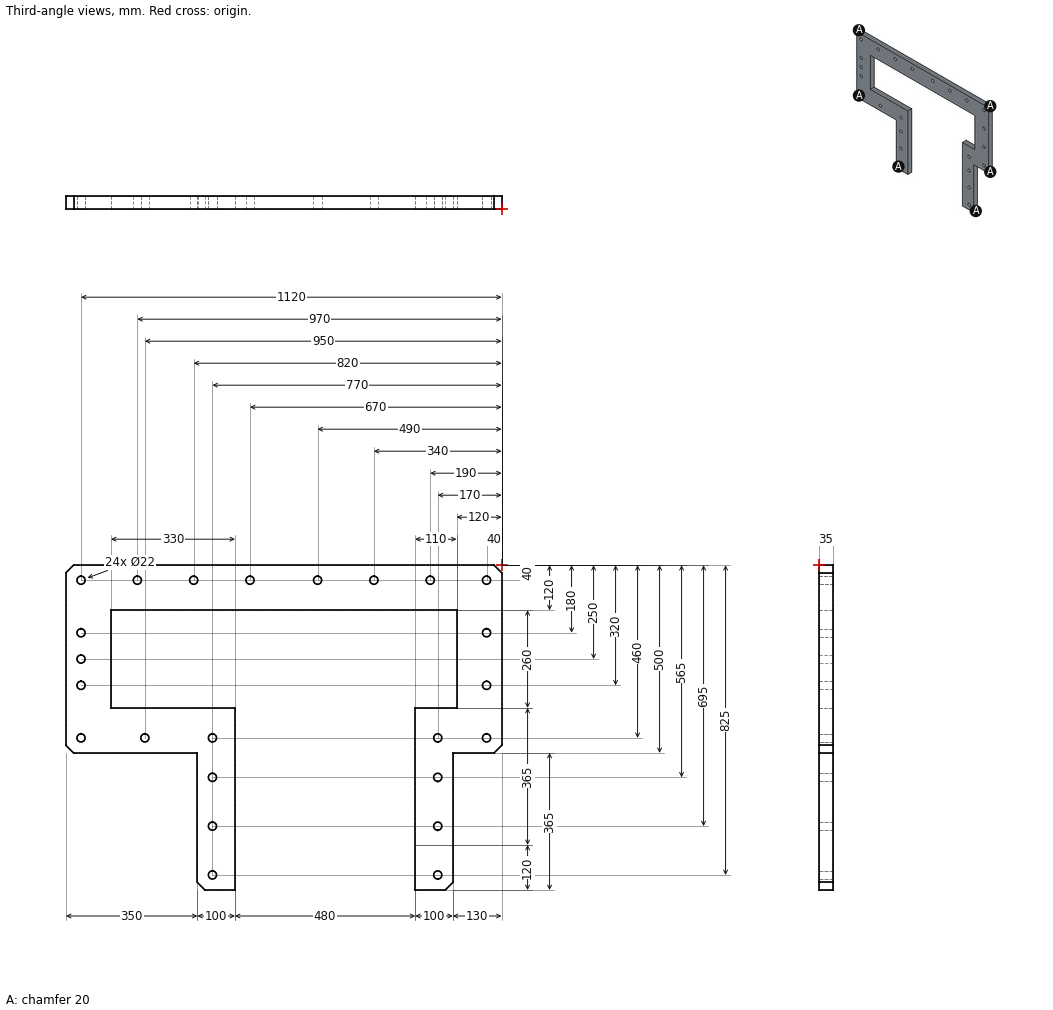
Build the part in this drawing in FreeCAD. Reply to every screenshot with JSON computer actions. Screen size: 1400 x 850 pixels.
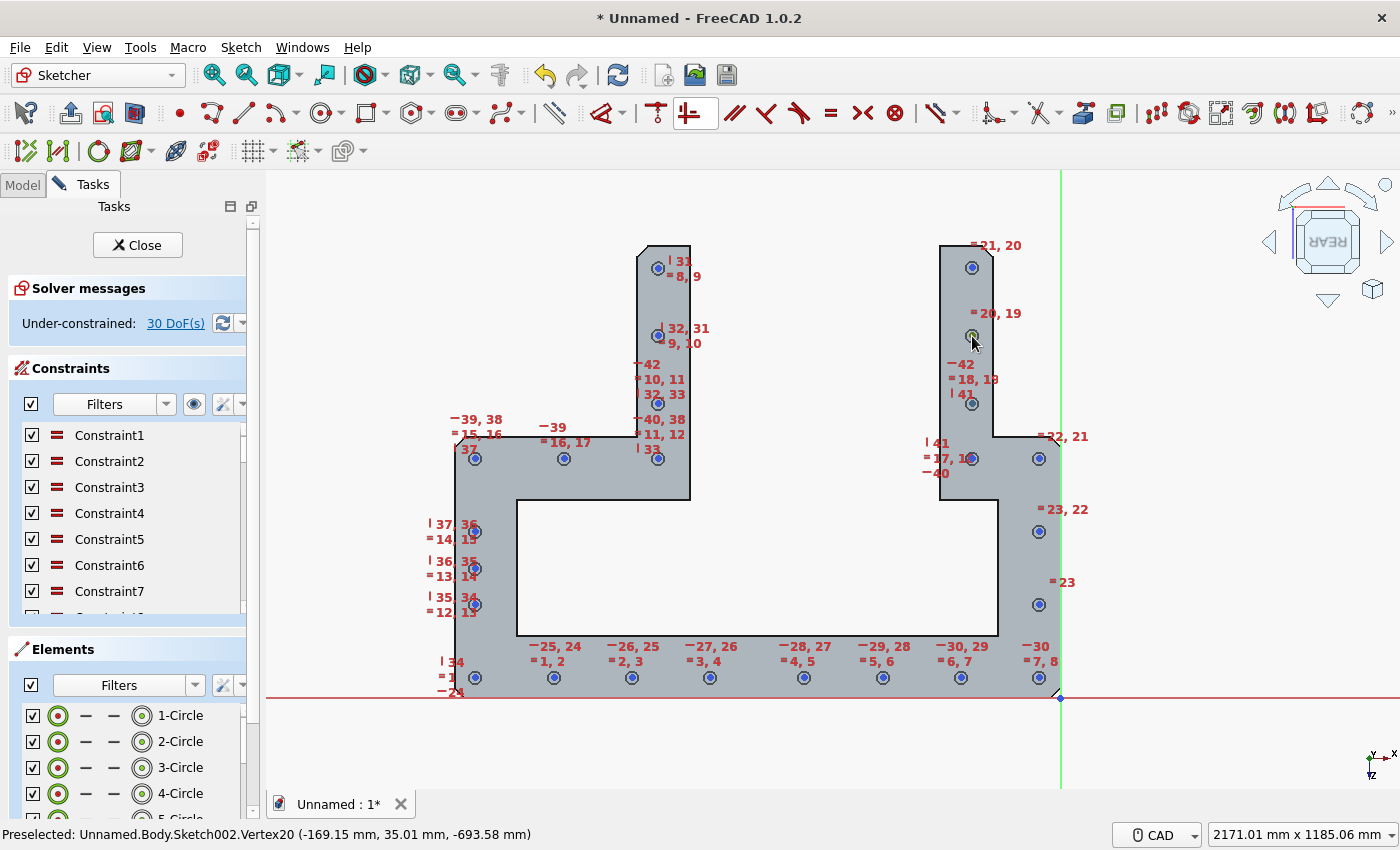
{"action": "key", "text": "v"}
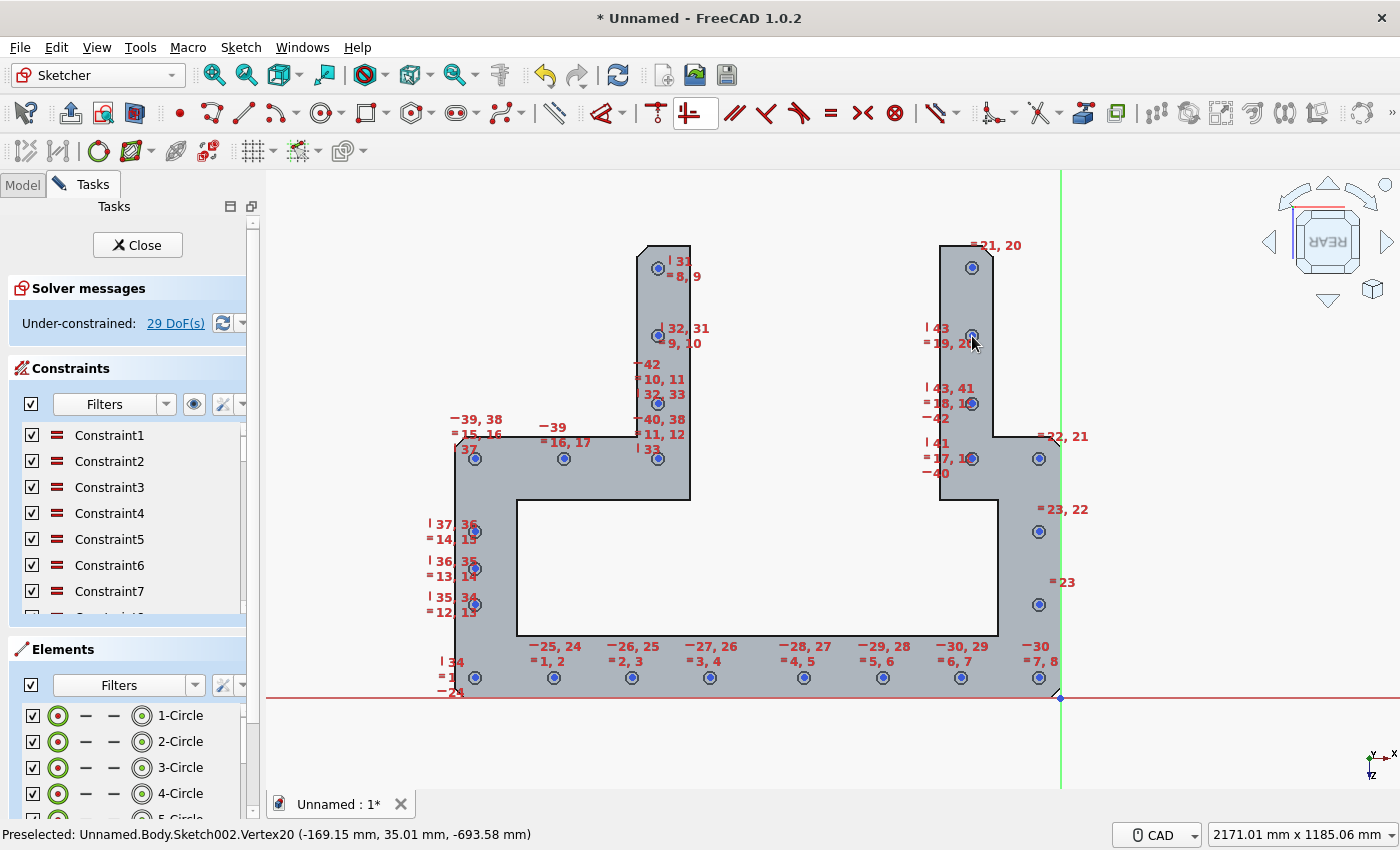
{"action": "left_click", "coordinate": [658, 336]}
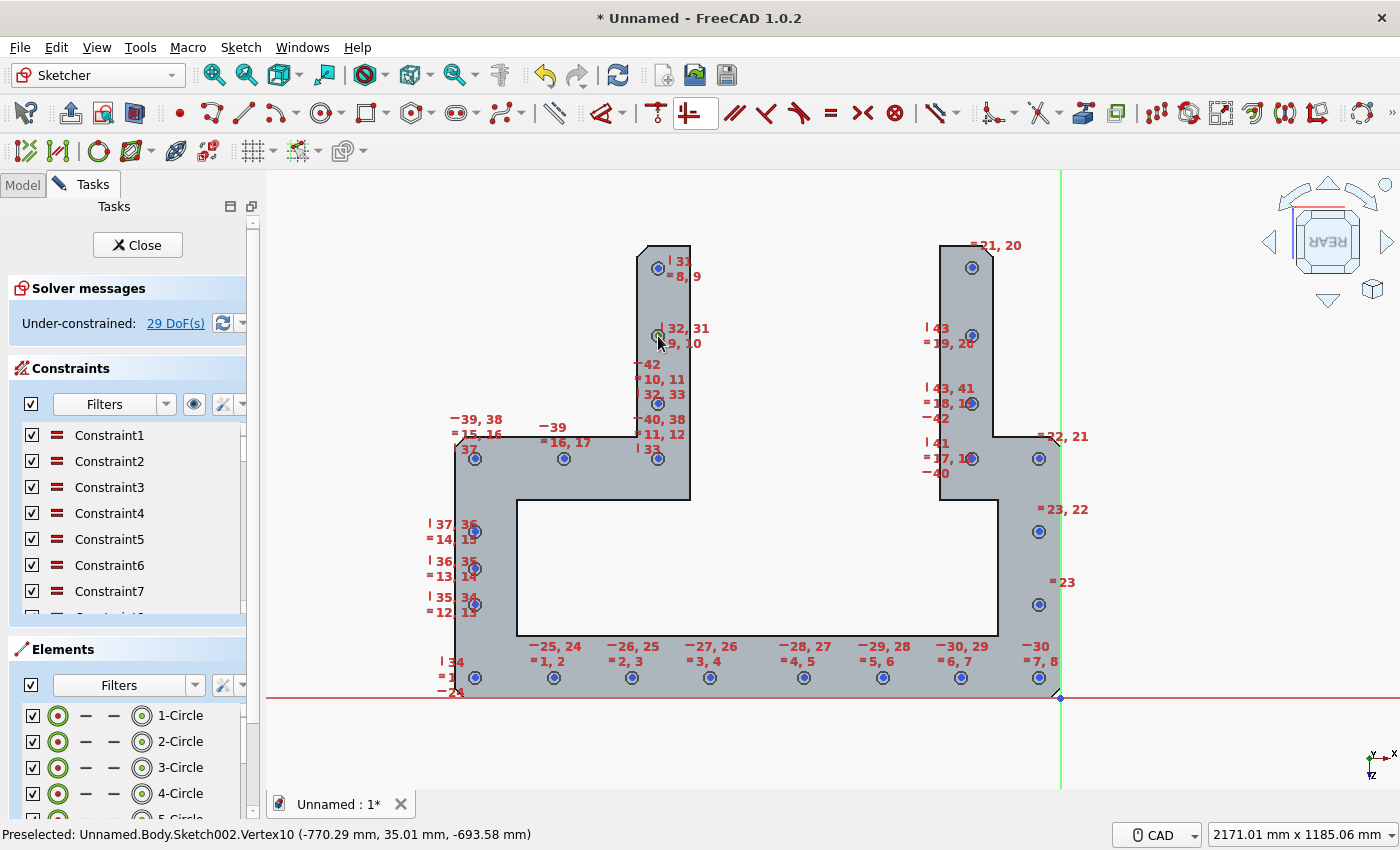
{"action": "left_click", "coordinate": [974, 338]}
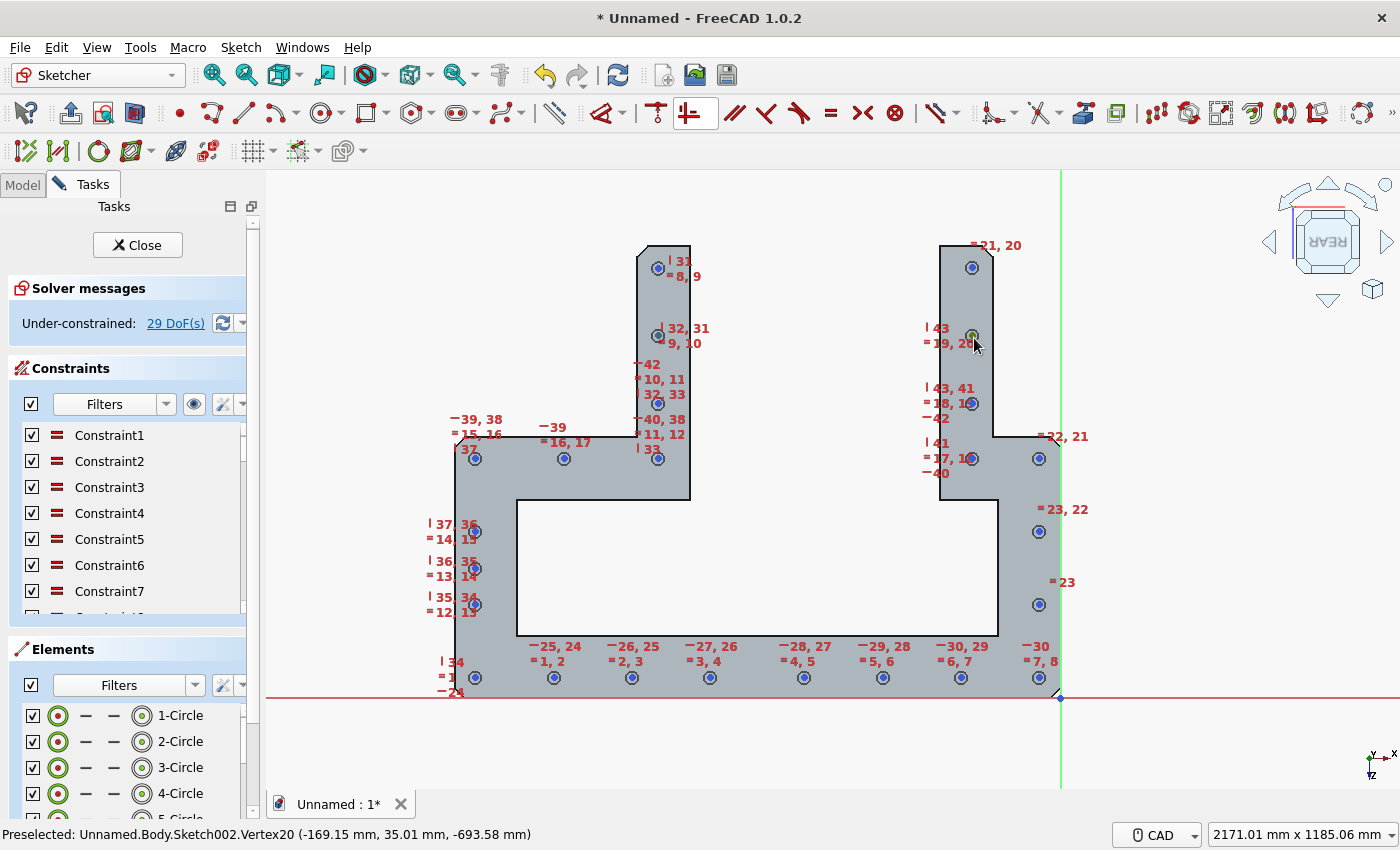
{"action": "key", "text": "h"}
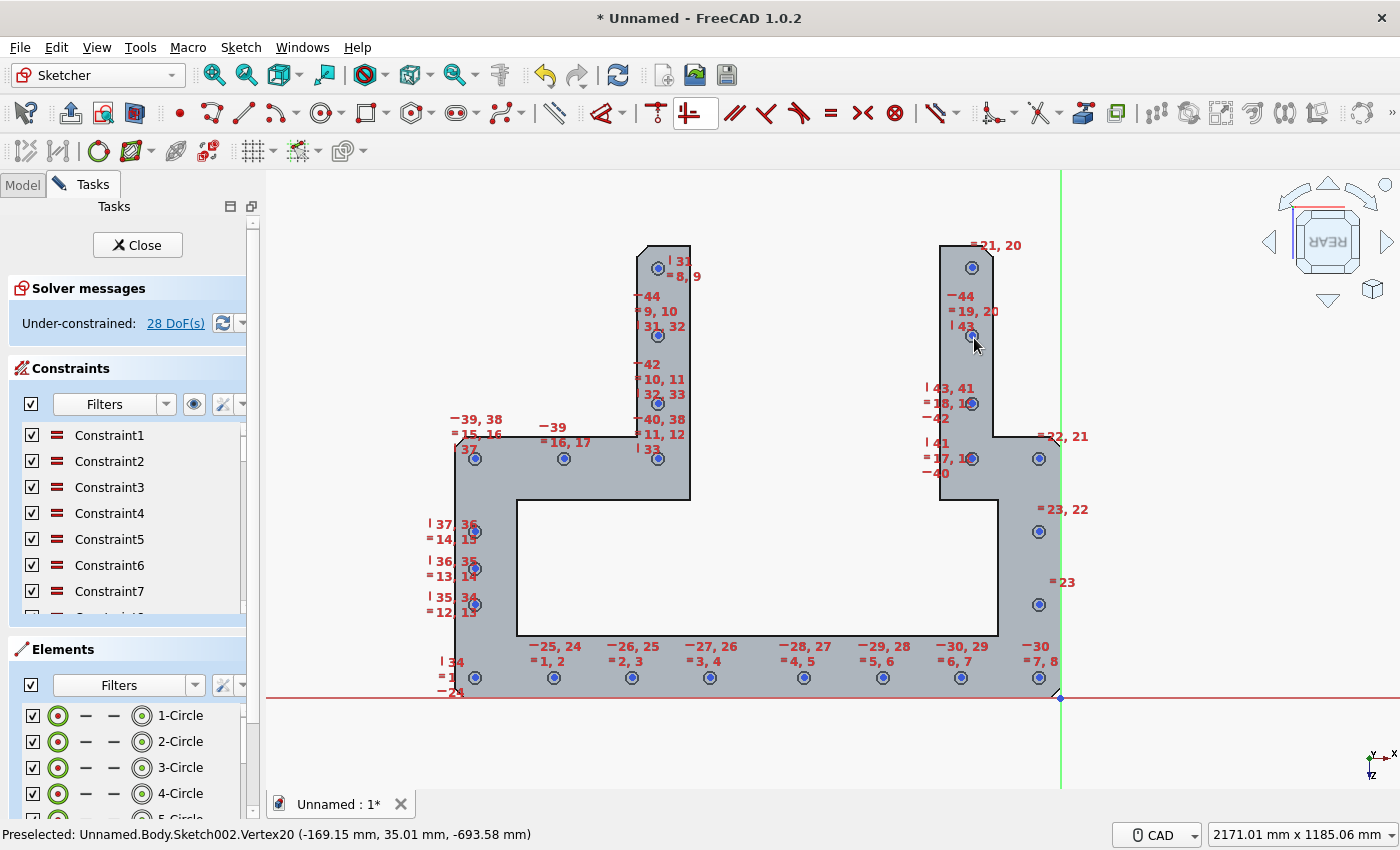
{"action": "left_click", "coordinate": [972, 336]}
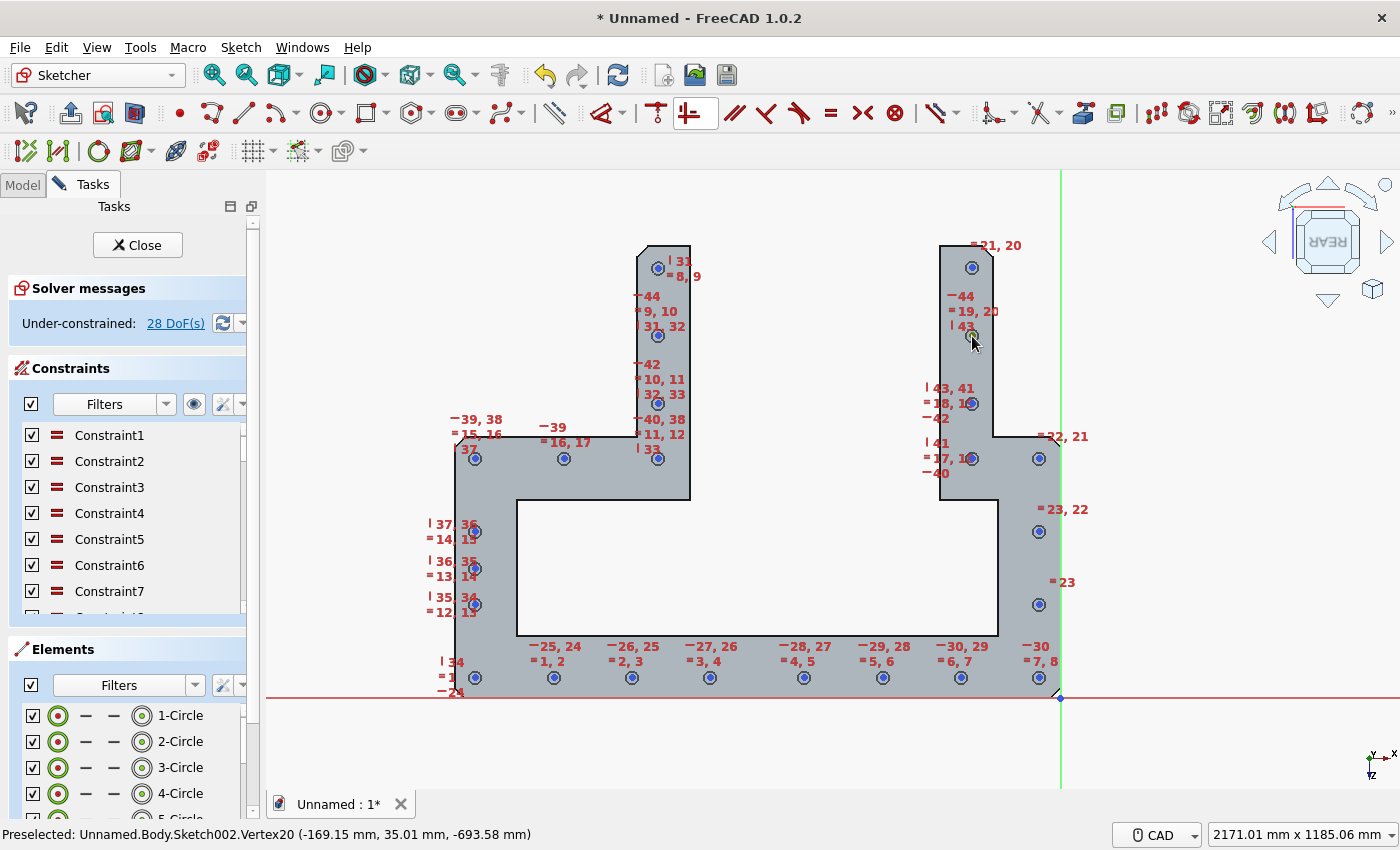
{"action": "left_click", "coordinate": [972, 268]}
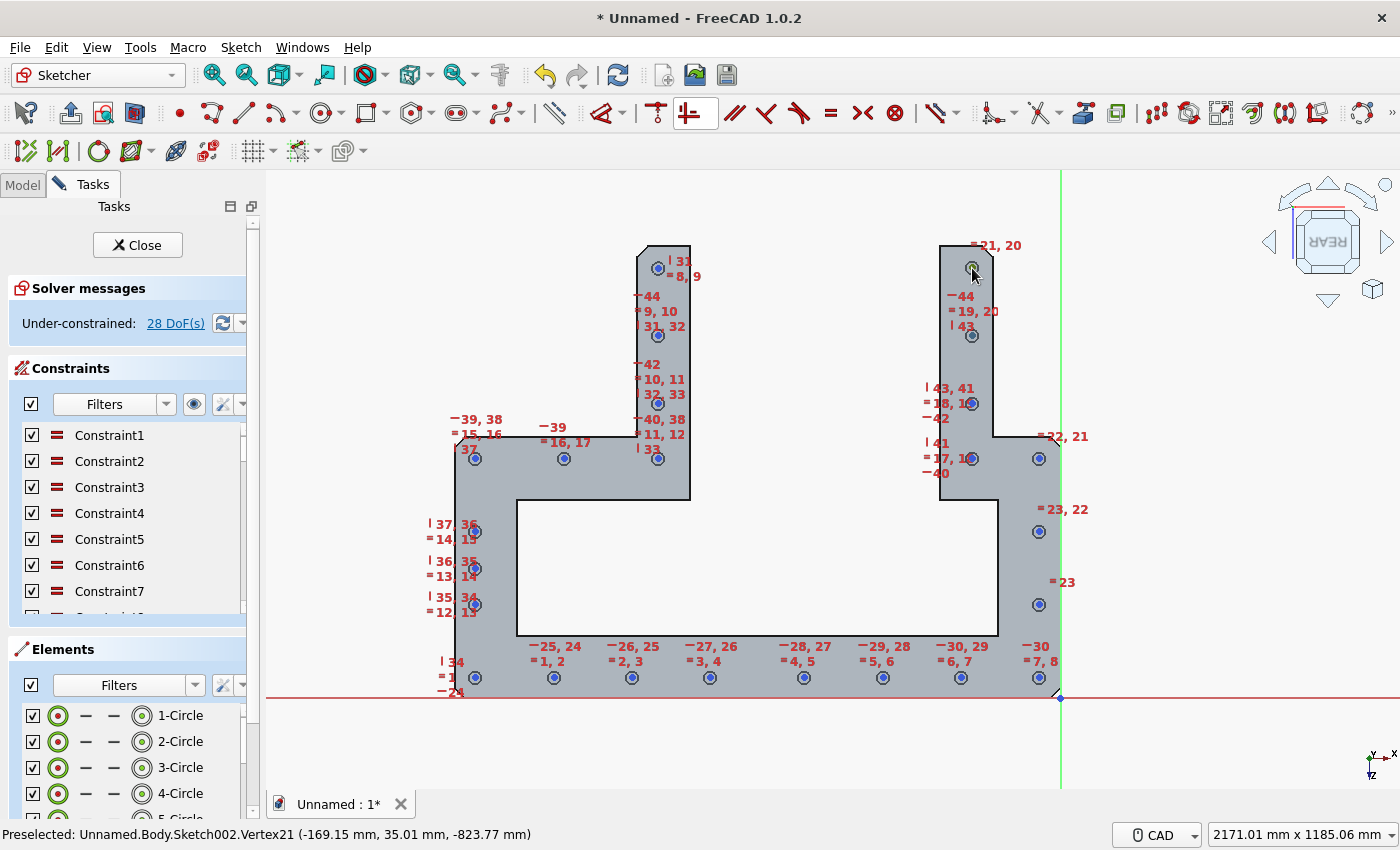
{"action": "key", "text": "v"}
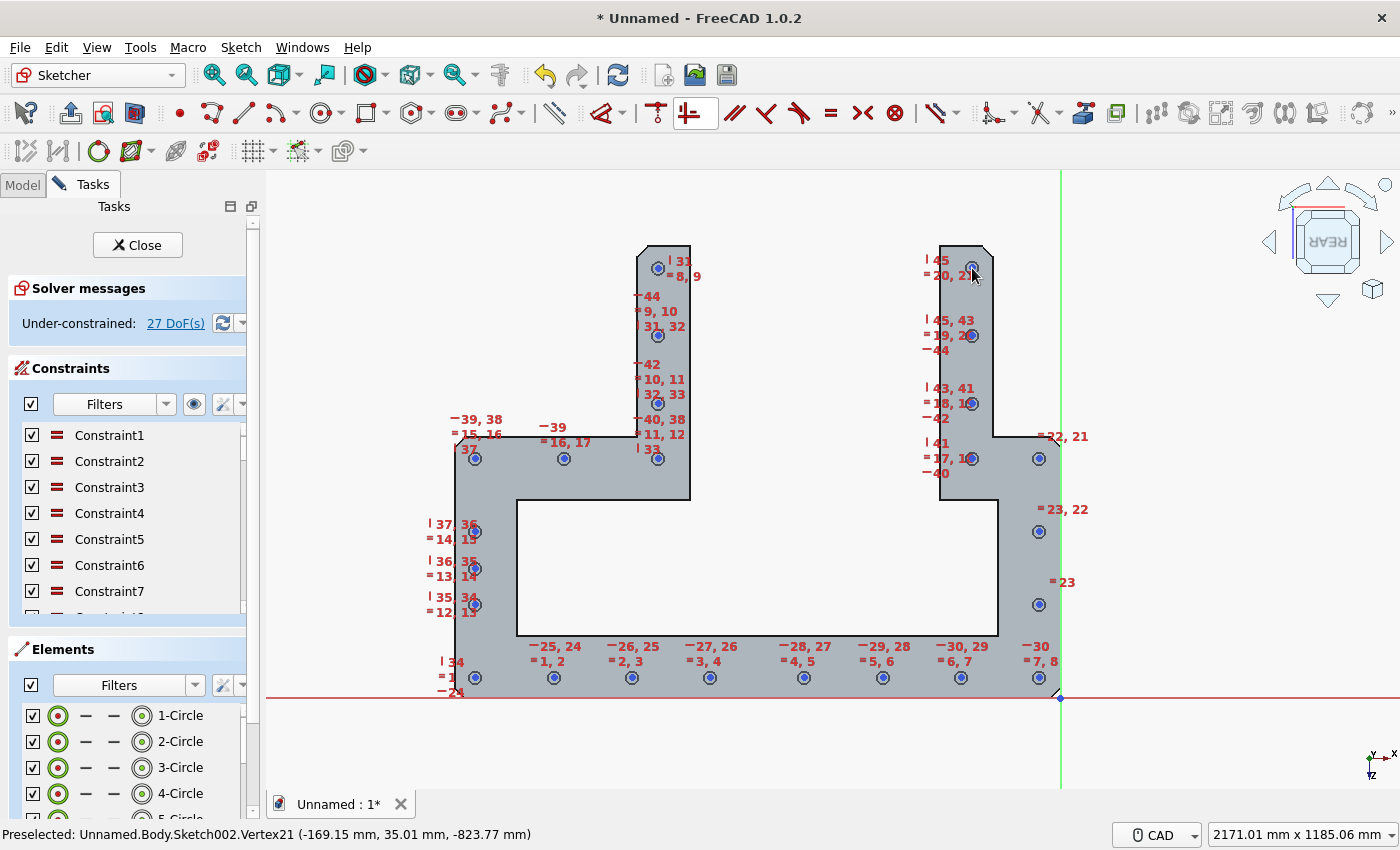
{"action": "left_click", "coordinate": [658, 269]}